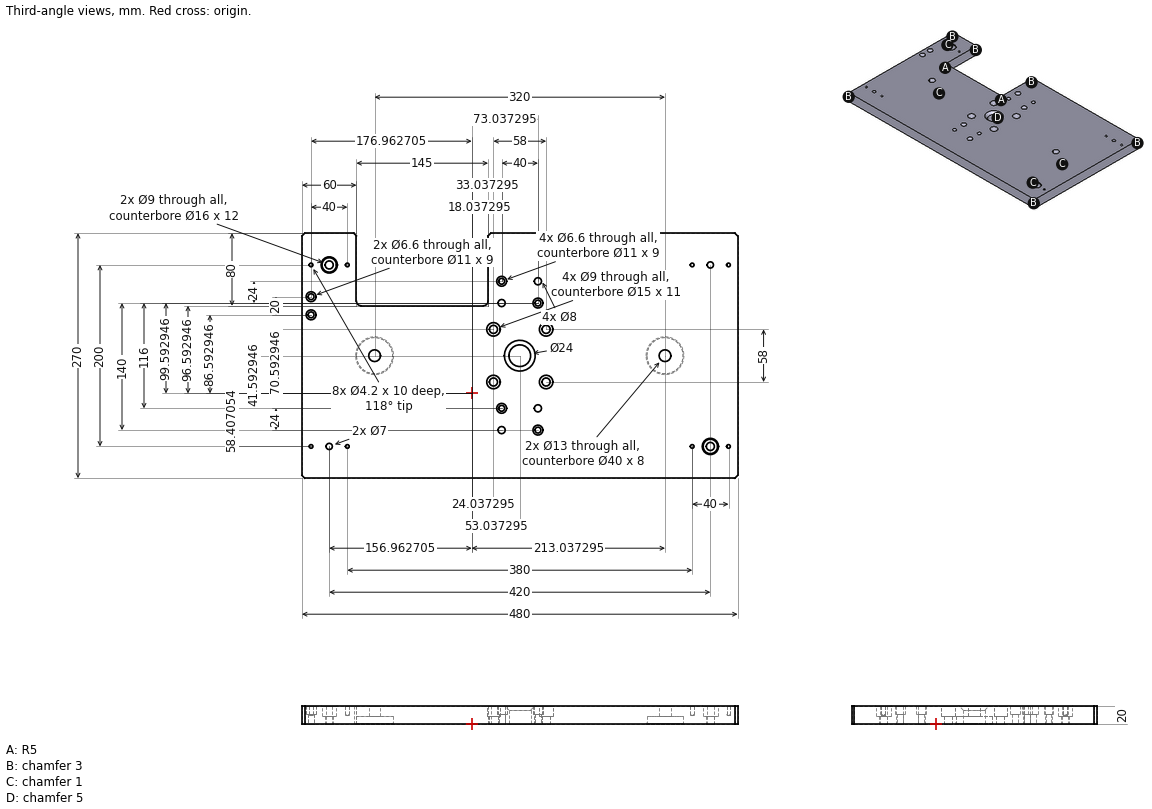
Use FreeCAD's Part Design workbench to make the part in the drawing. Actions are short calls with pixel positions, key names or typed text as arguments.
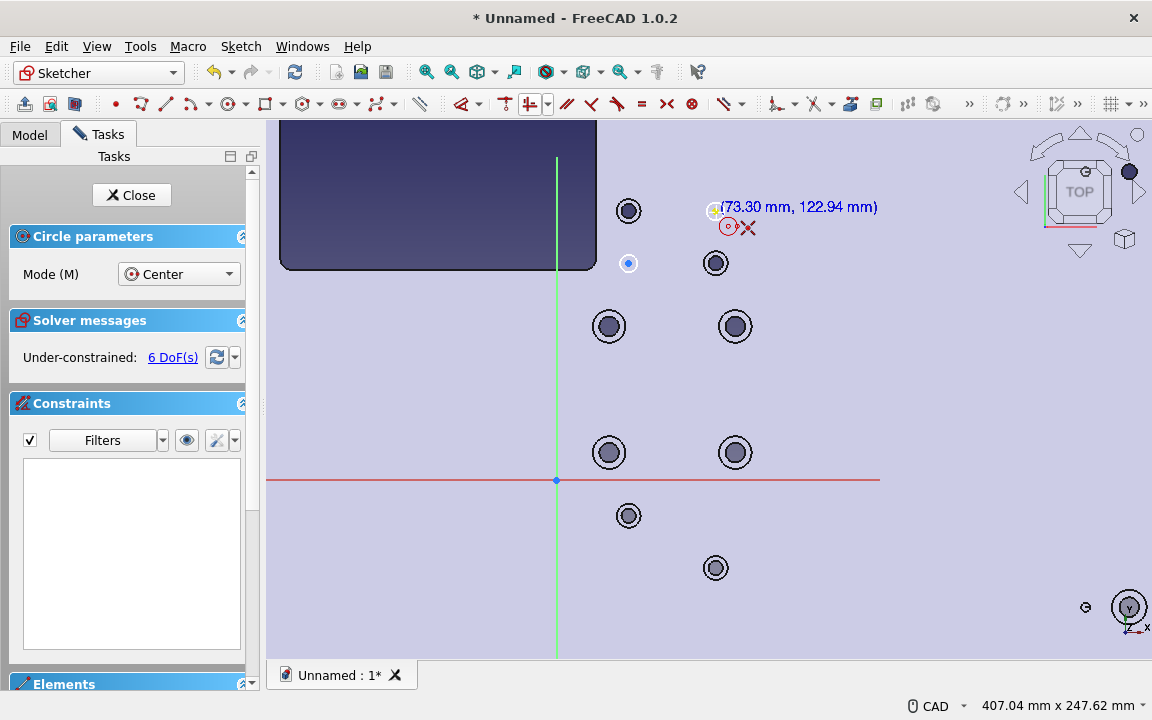
scroll(629, 568, up, 5)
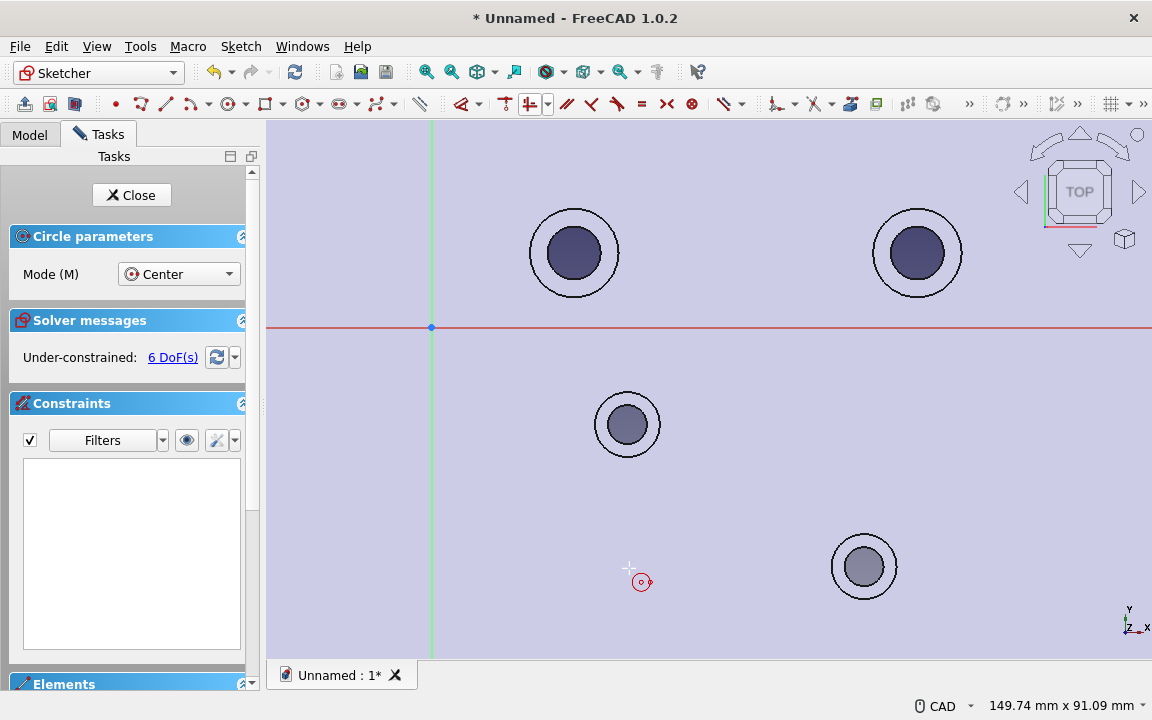
click(627, 567)
click(644, 550)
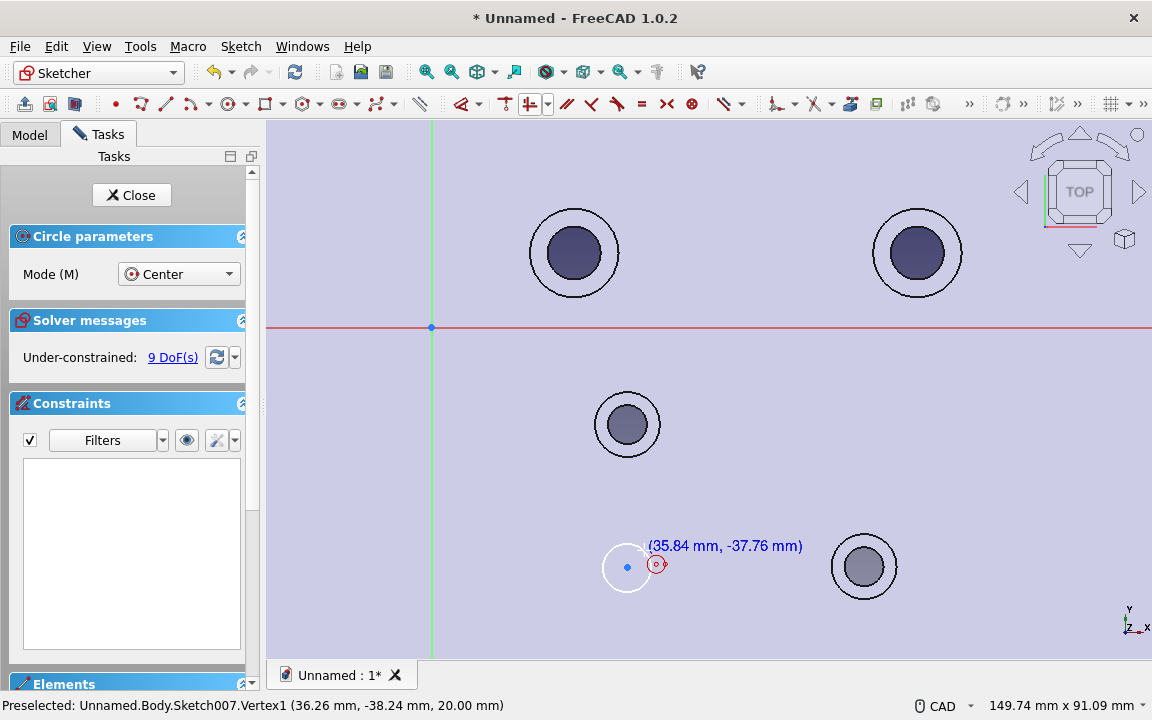
click(864, 425)
click(881, 408)
key(Escape)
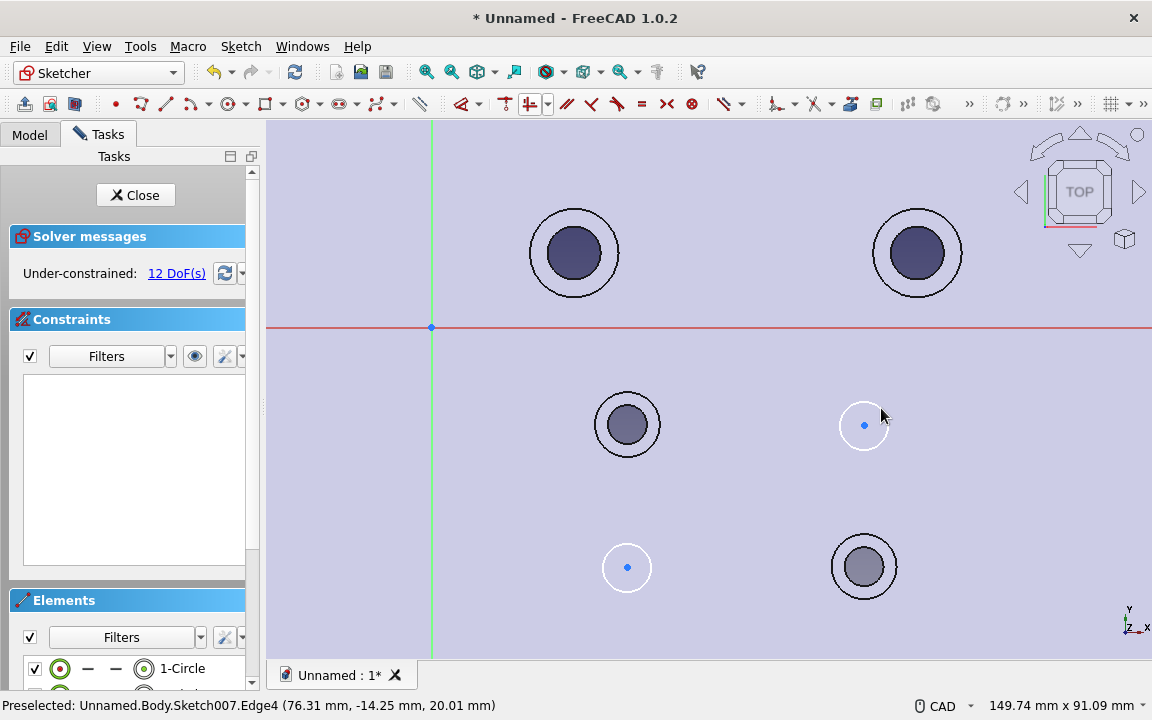
scroll(629, 569, down, 5)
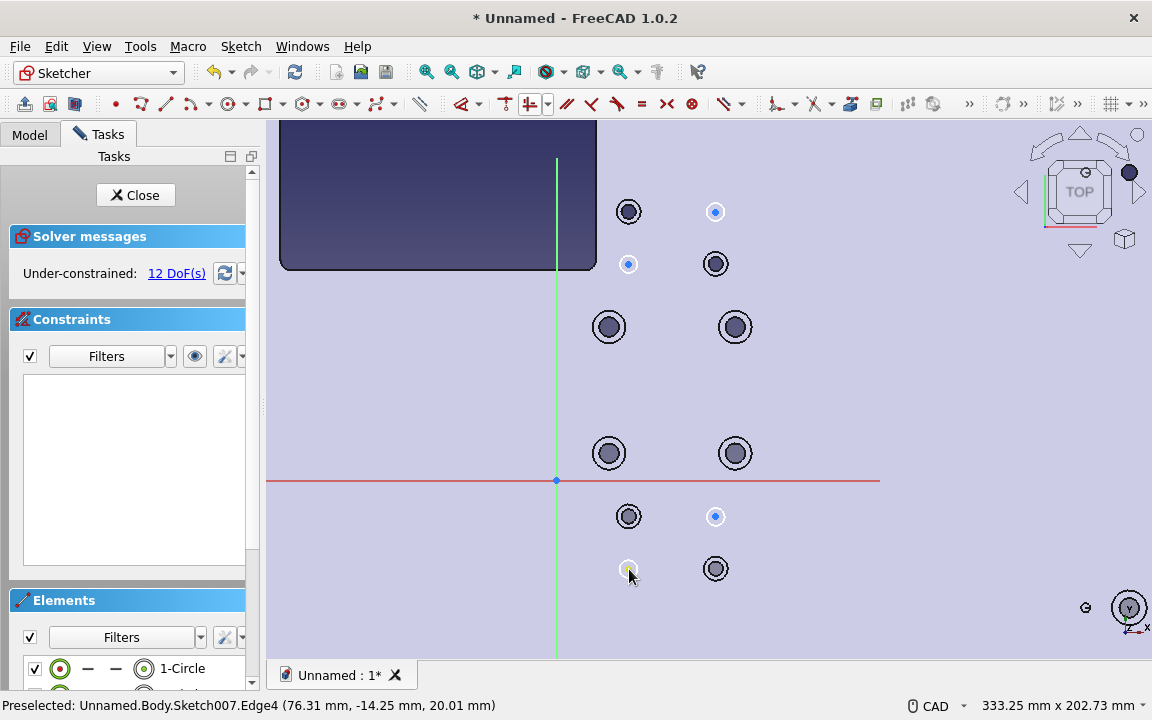
scroll(722, 206, up, 3)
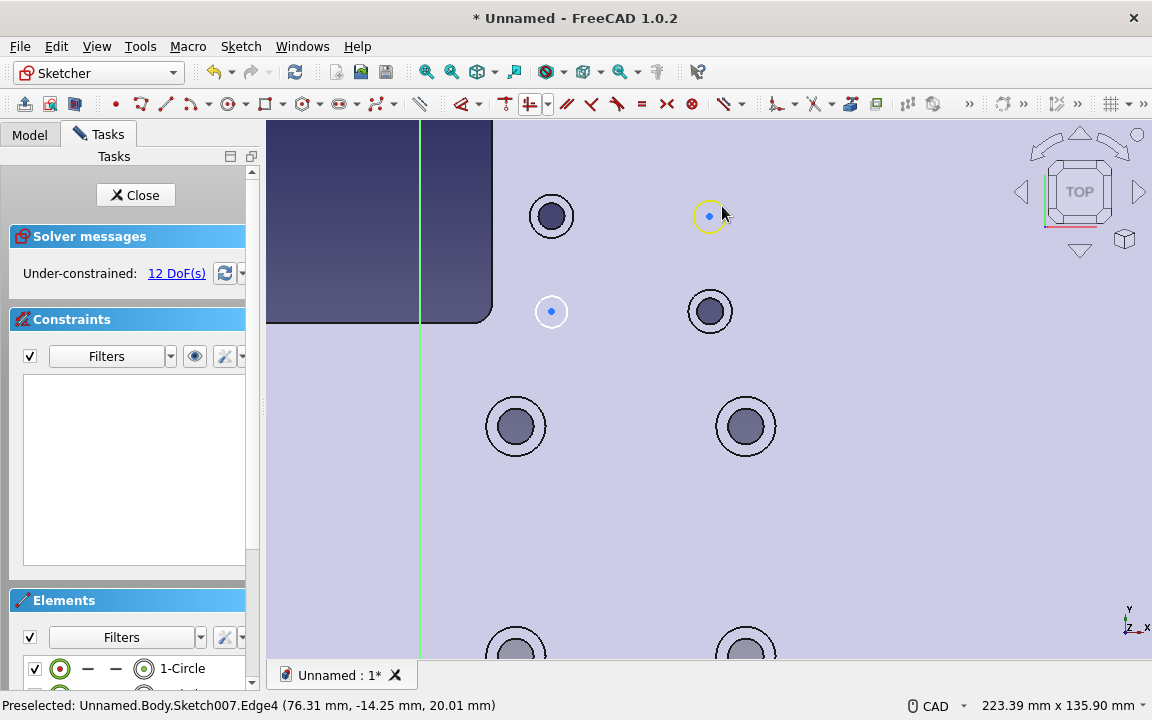
click(721, 205)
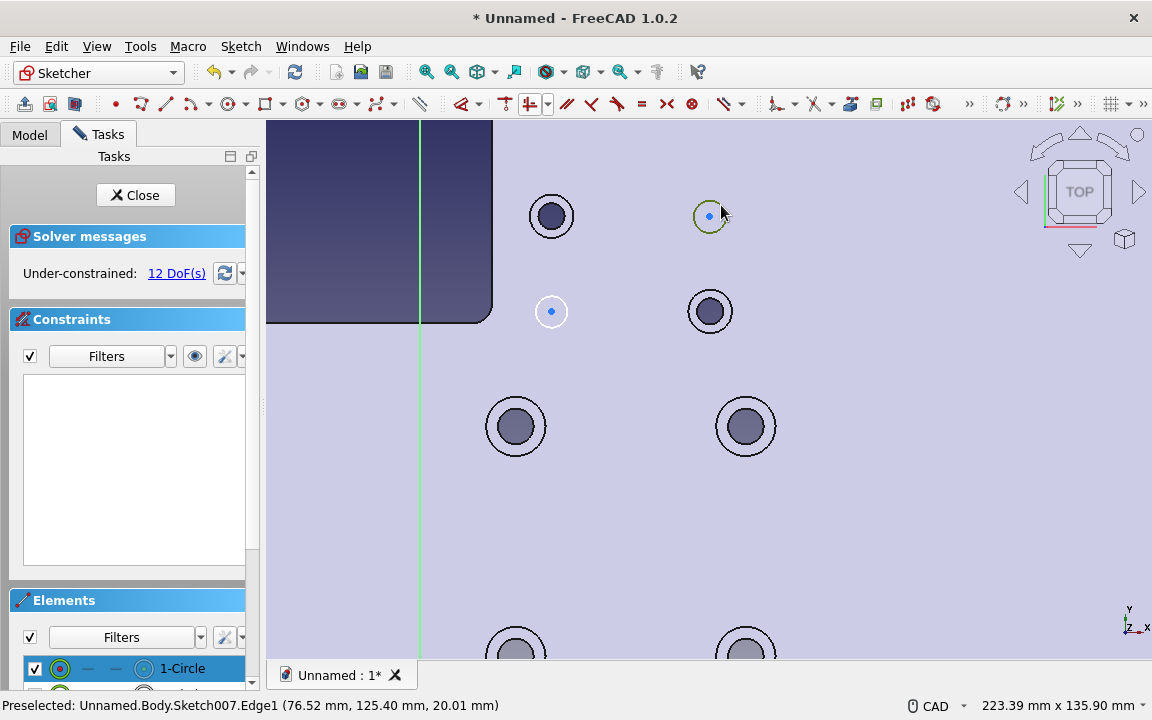
click(563, 301)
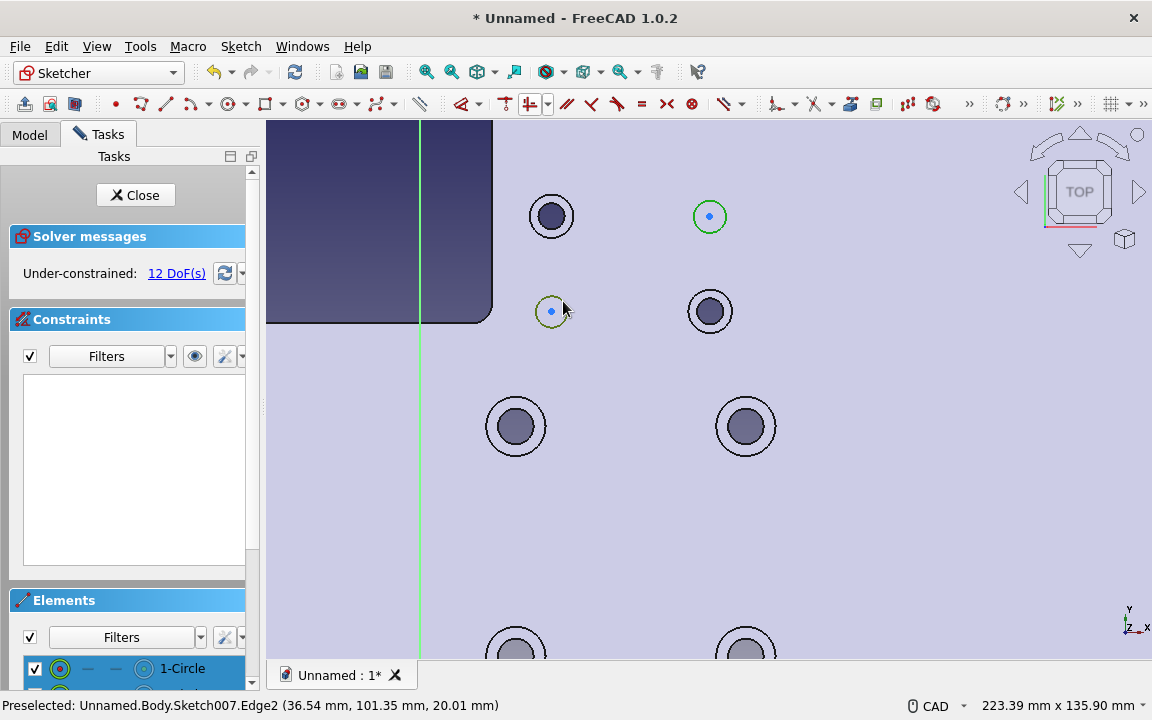
scroll(722, 205, down, 3)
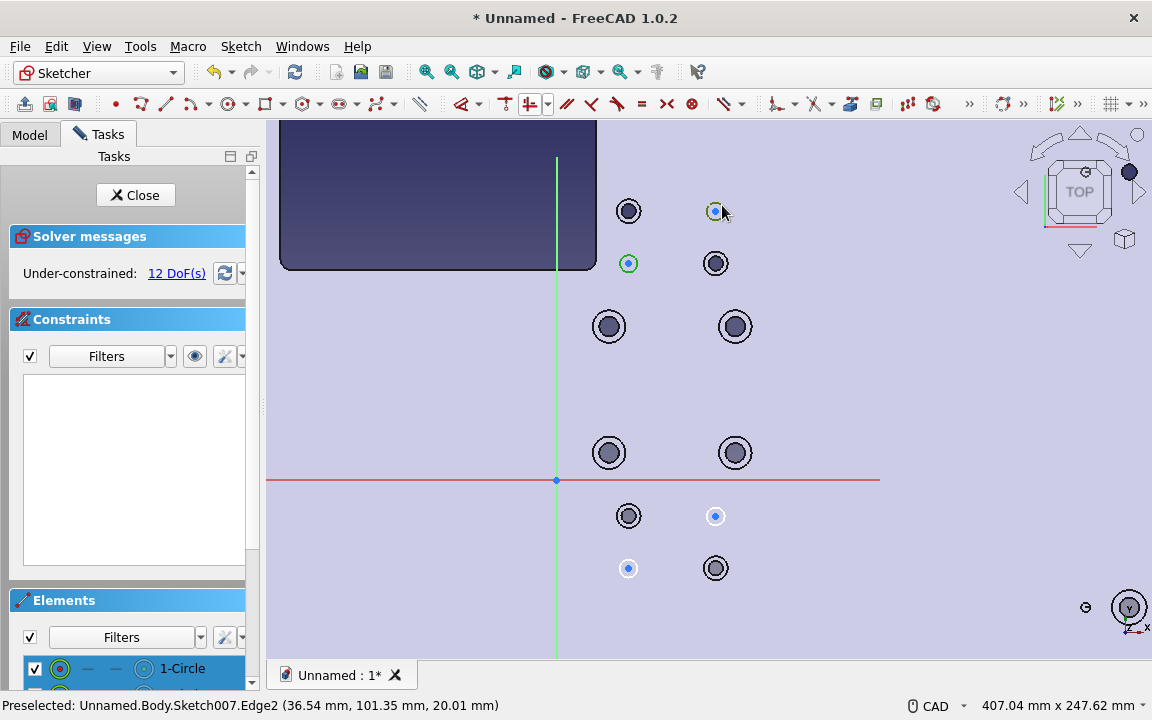
scroll(635, 562, up, 3)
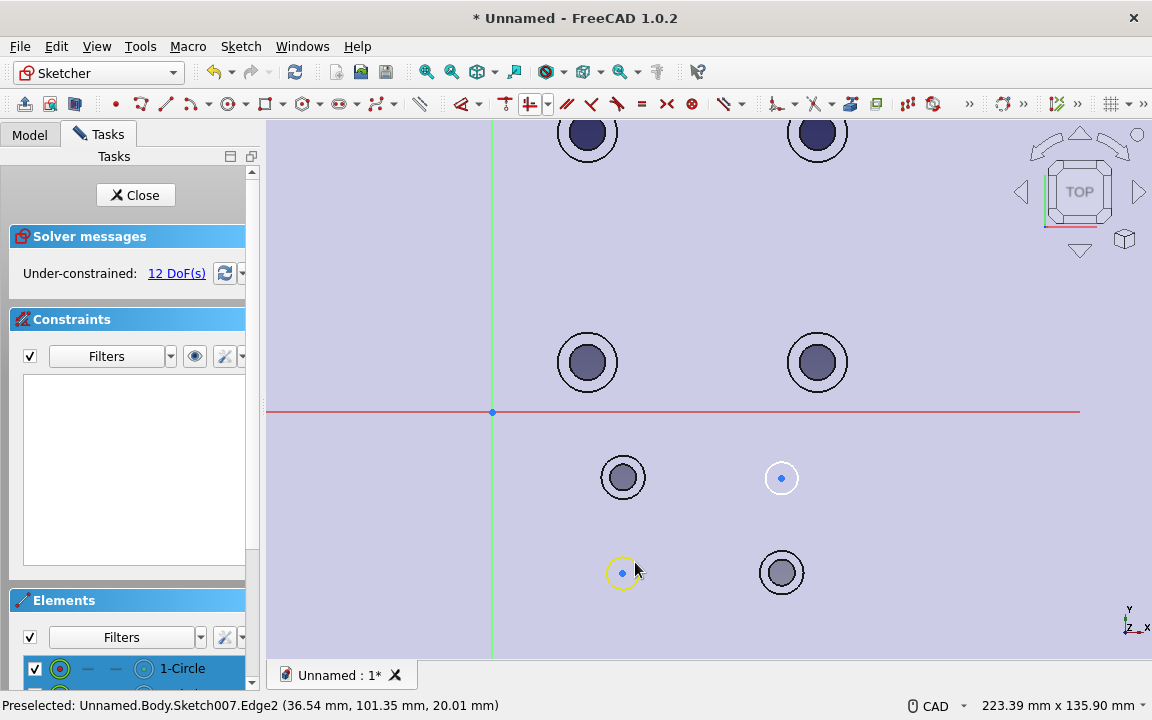
click(634, 562)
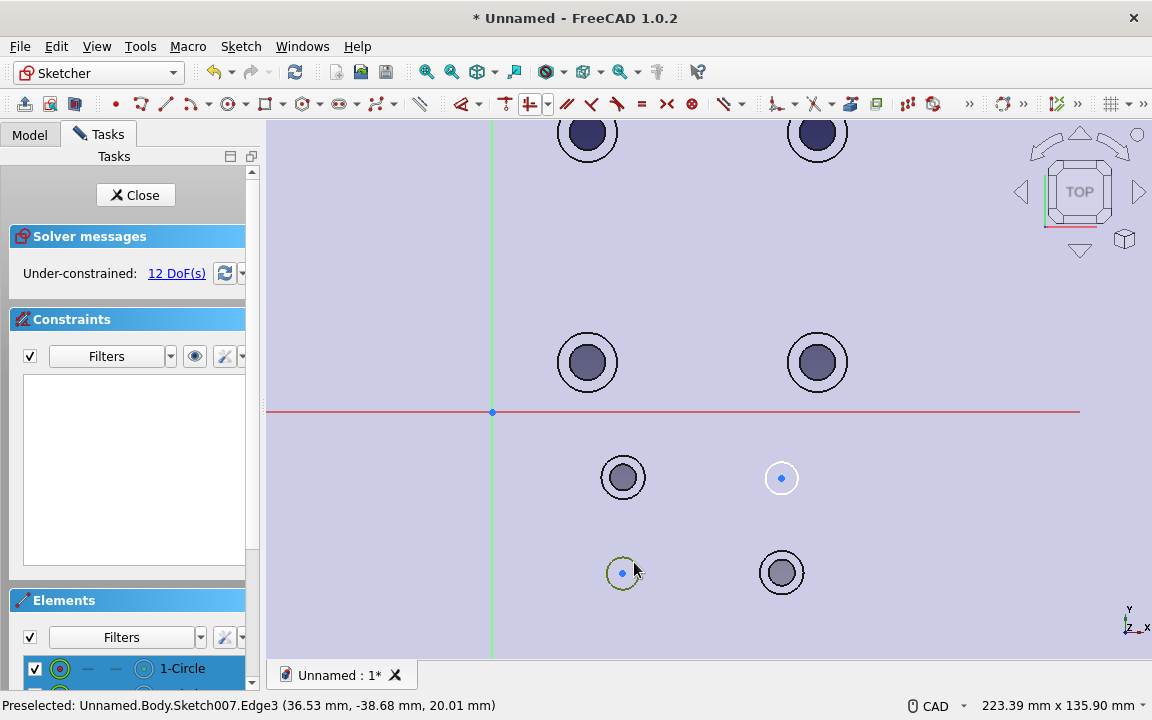
click(793, 467)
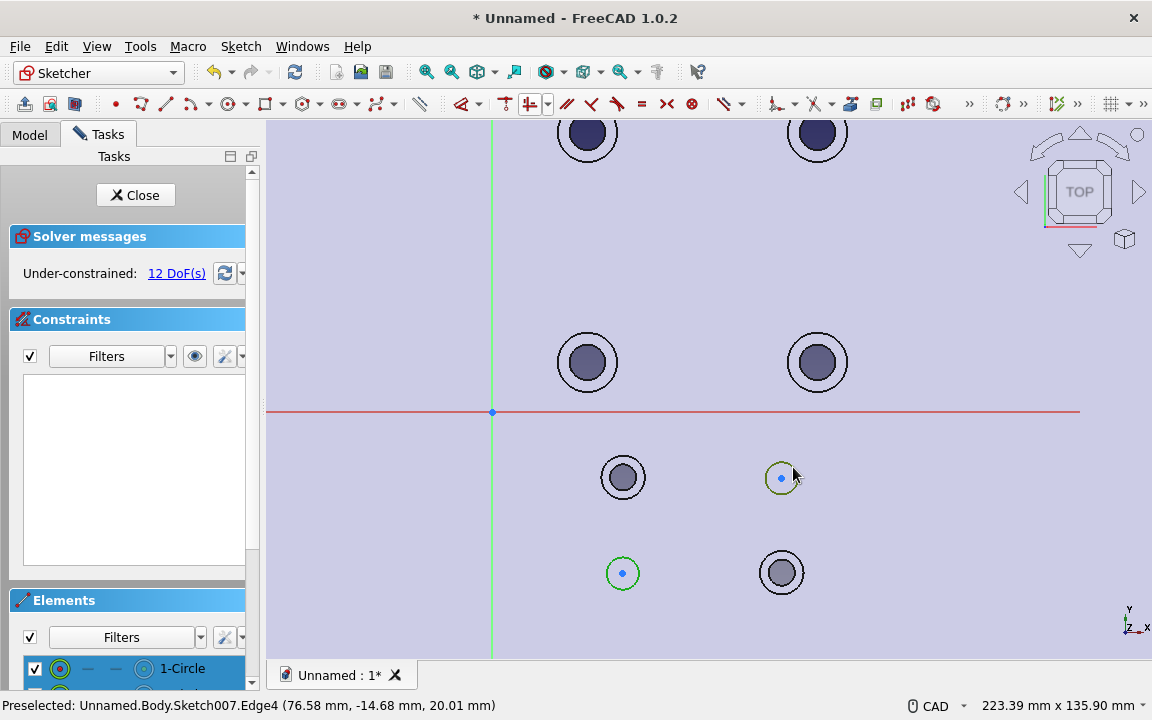
key(e)